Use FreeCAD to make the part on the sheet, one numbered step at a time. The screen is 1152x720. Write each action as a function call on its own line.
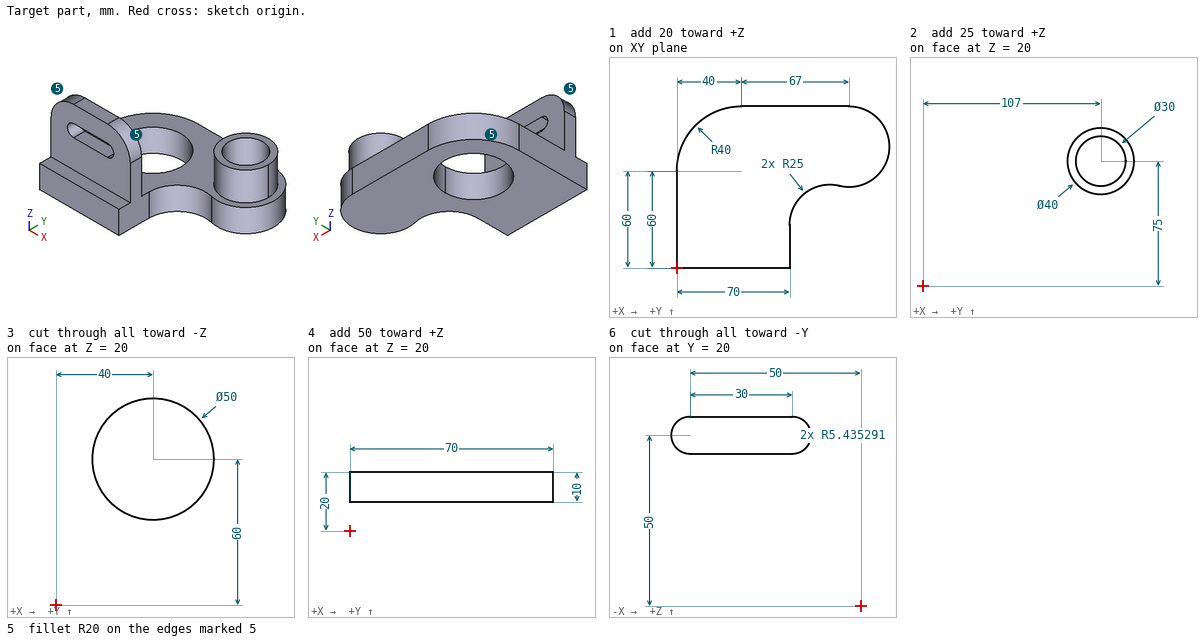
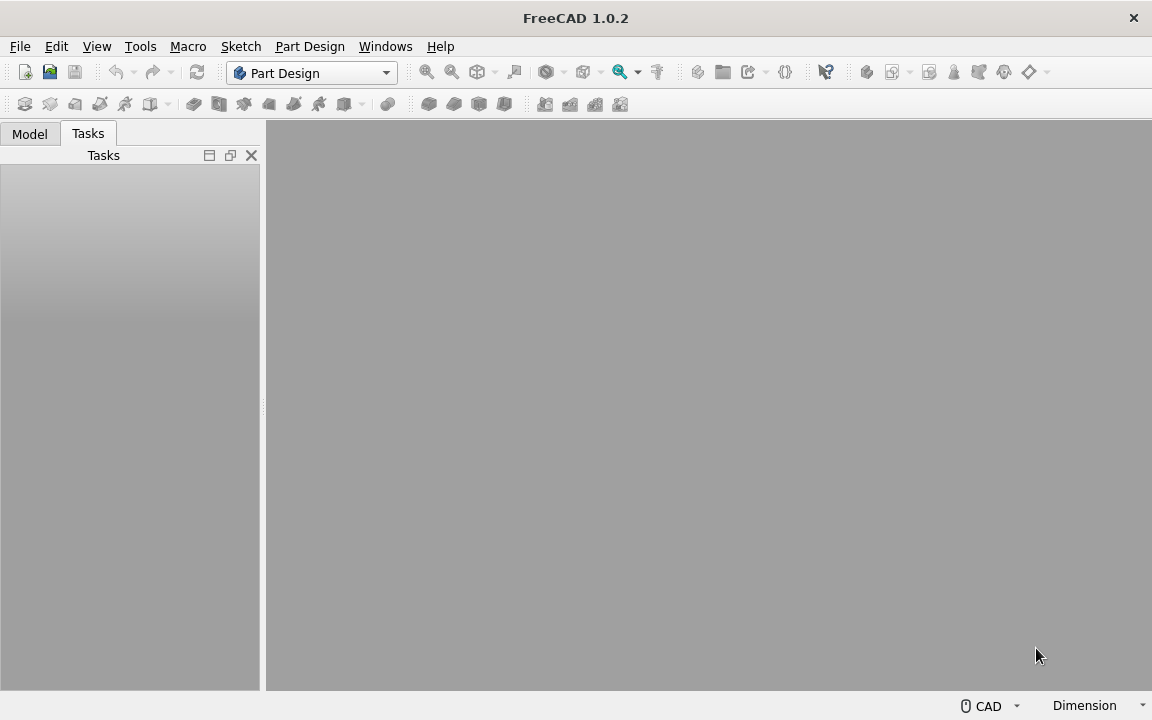
click(25, 72)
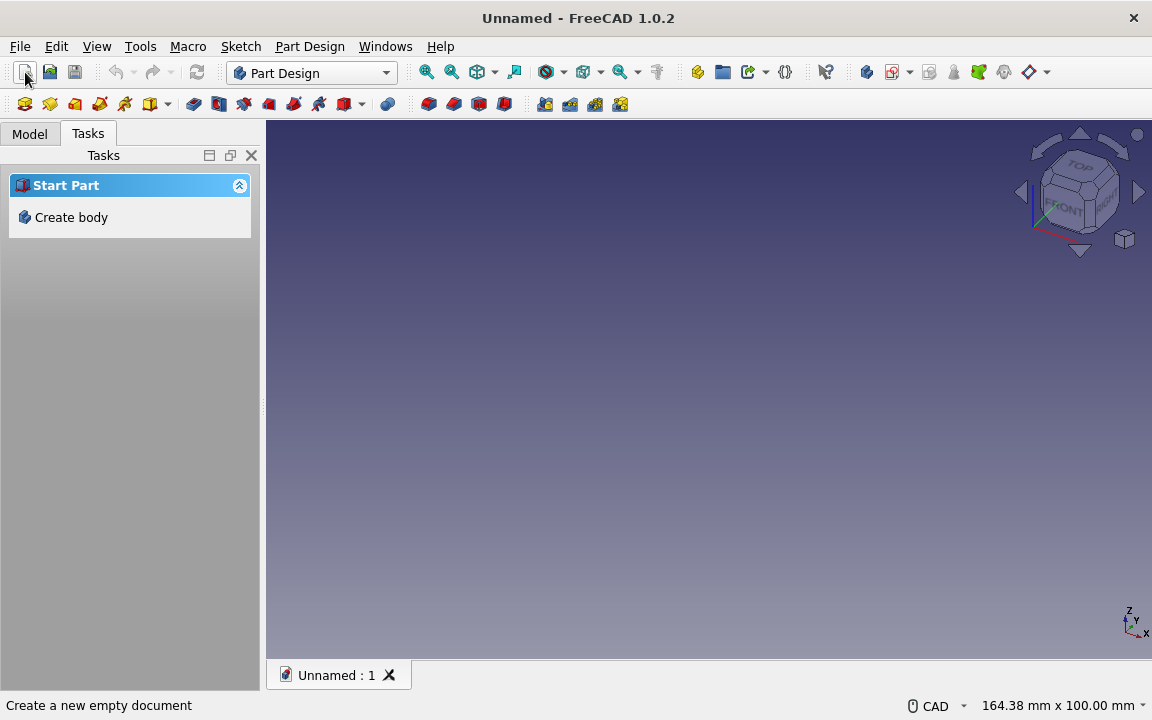
click(892, 72)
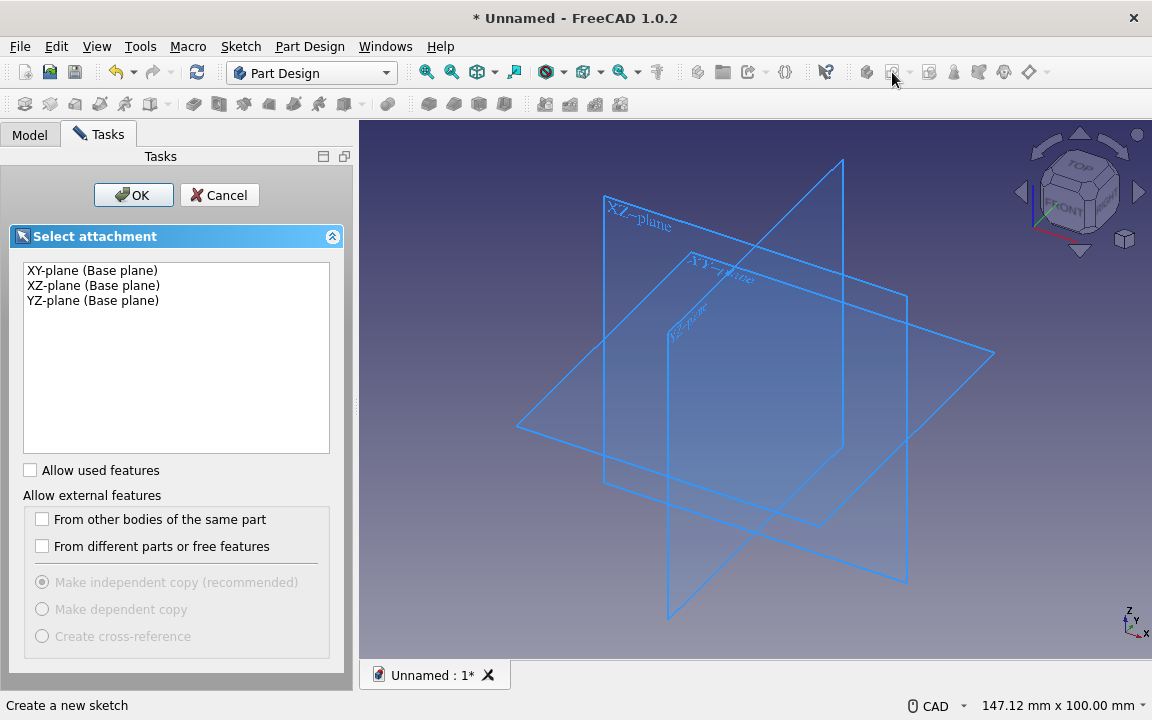
click(84, 270)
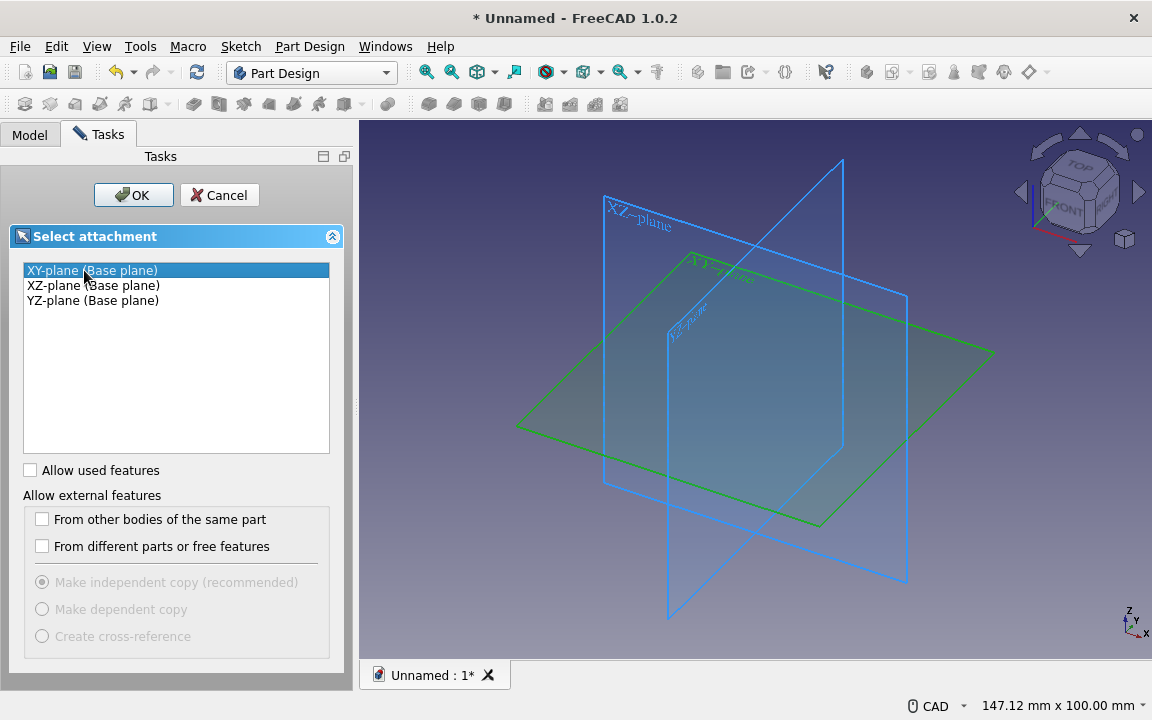
click(134, 195)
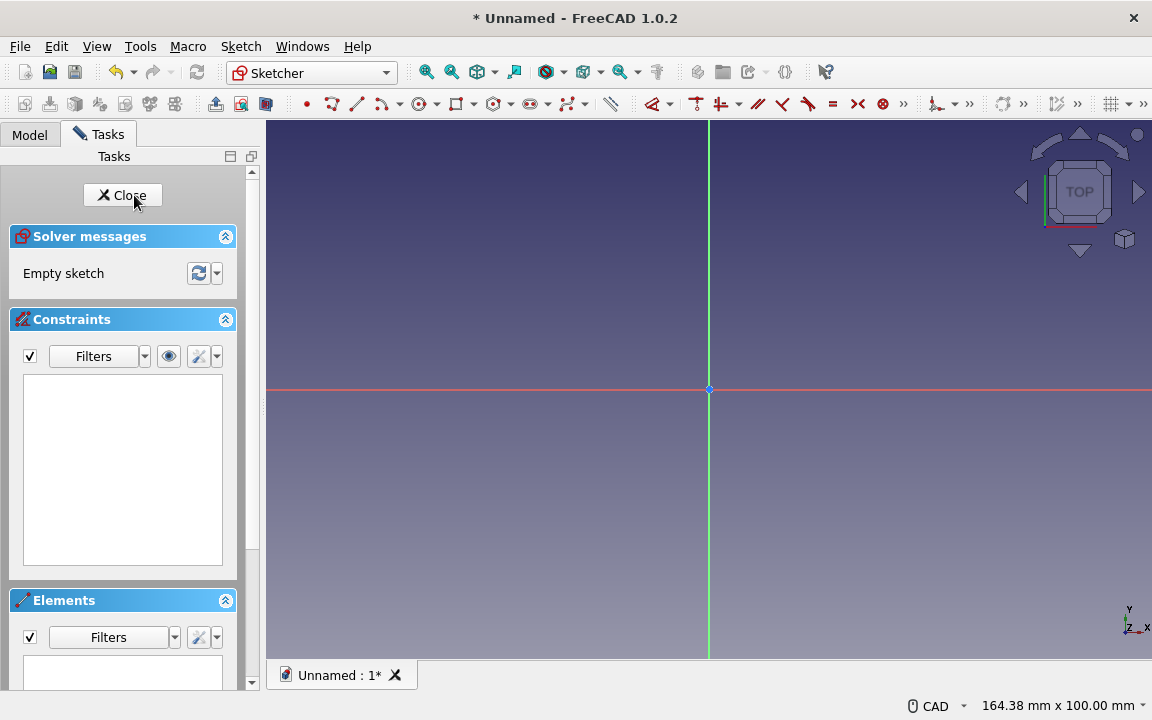
scroll(294, 631, down, 3)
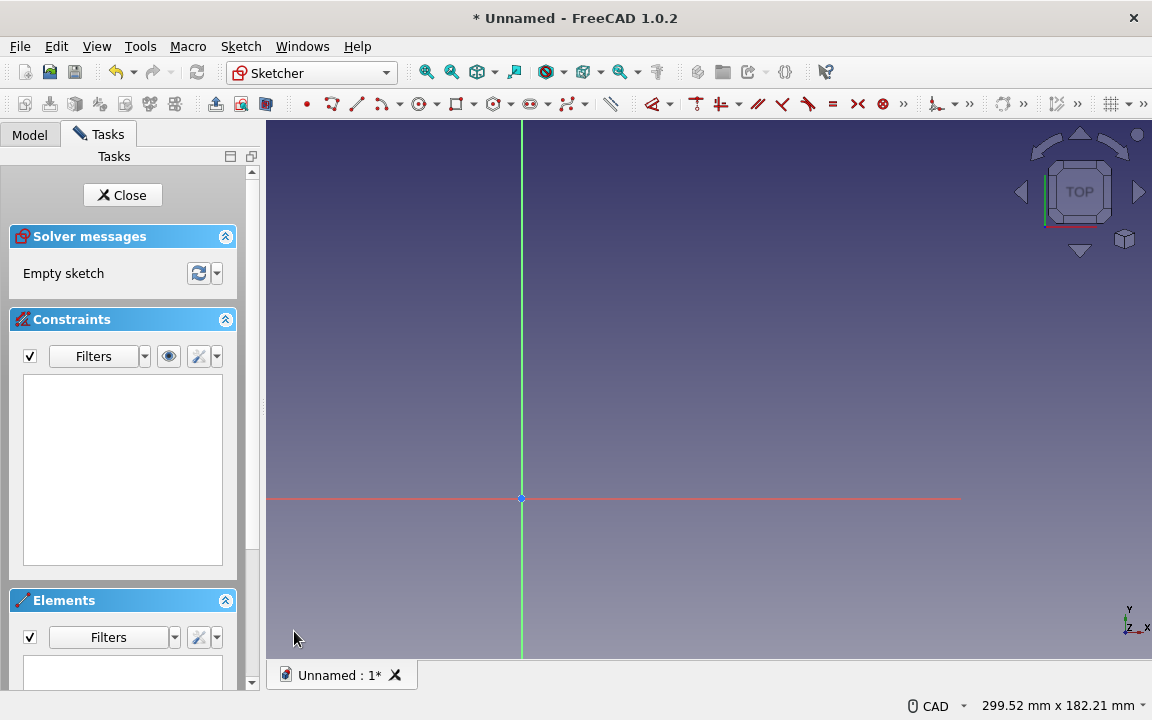
click(357, 104)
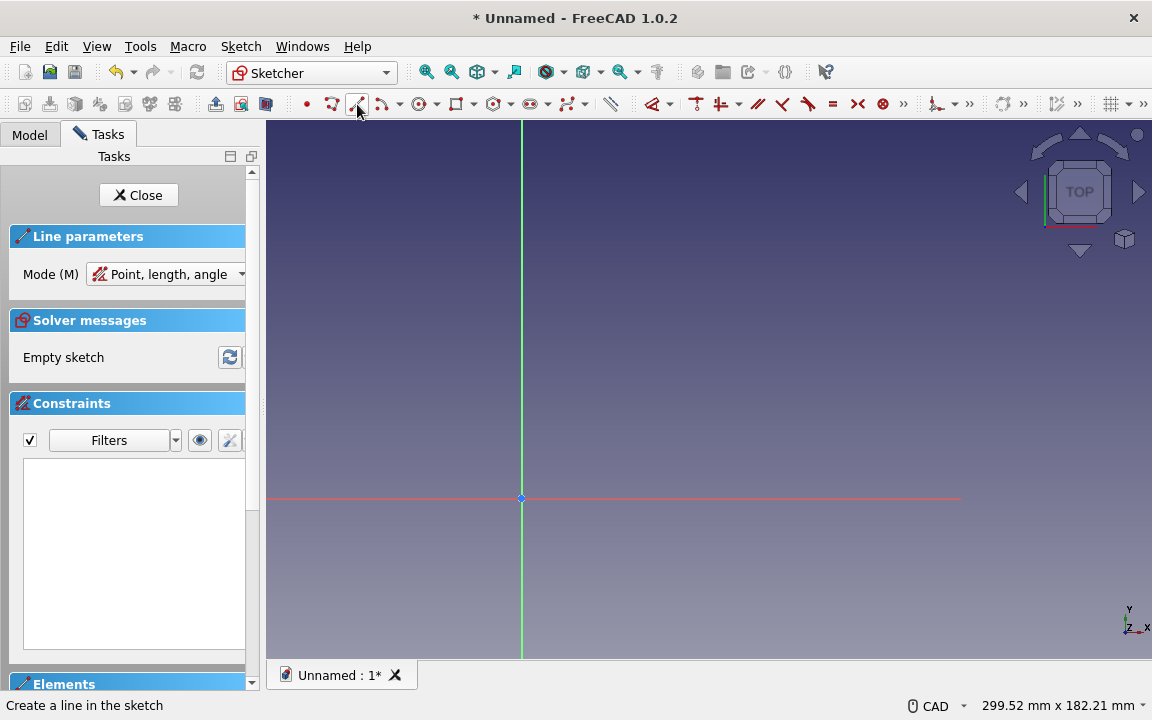
click(838, 203)
click(640, 203)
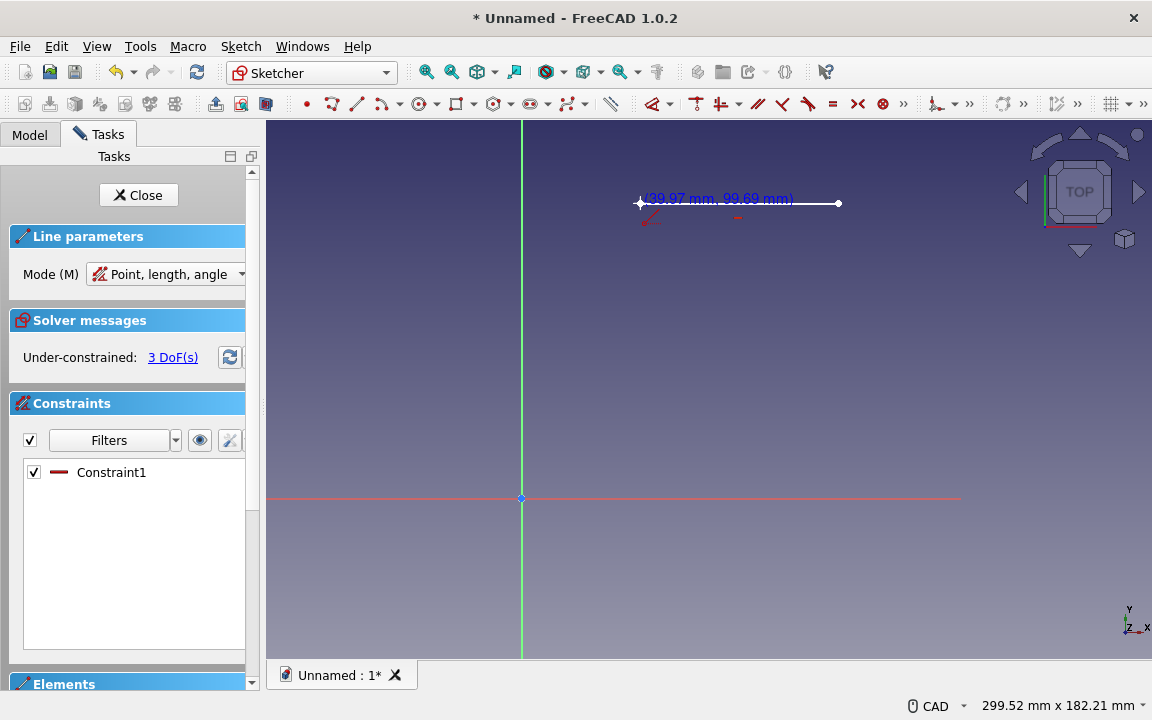
click(332, 104)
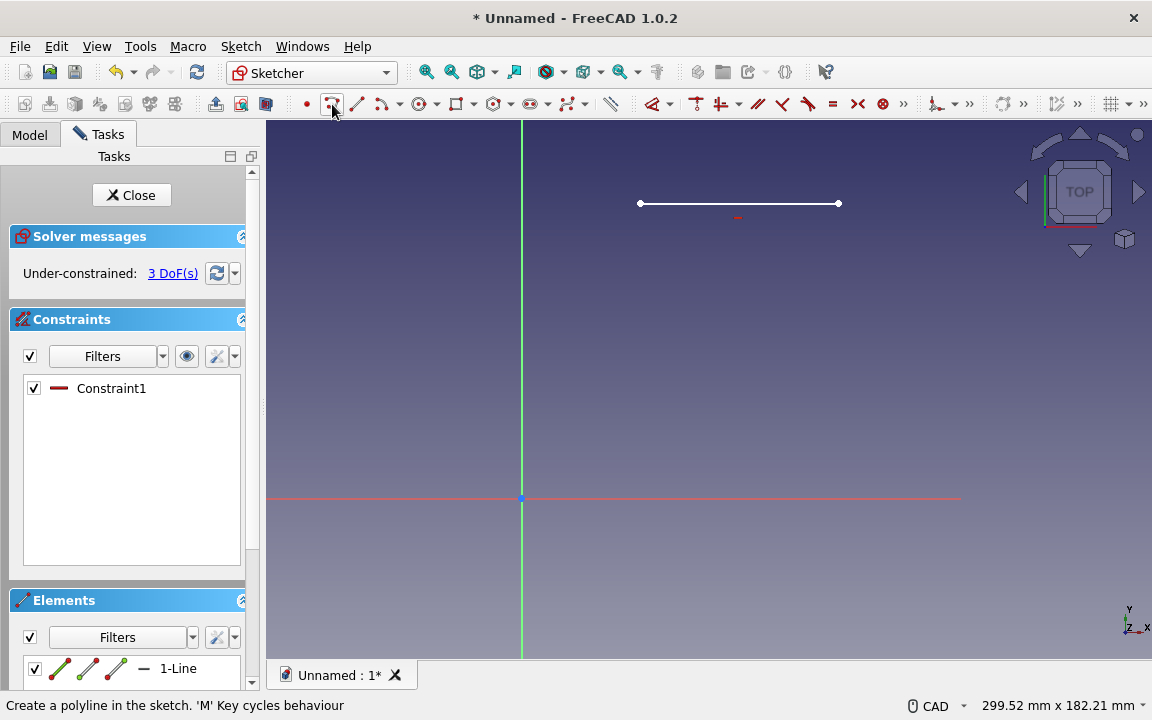
click(522, 321)
click(522, 499)
click(729, 490)
click(729, 421)
right_click(729, 421)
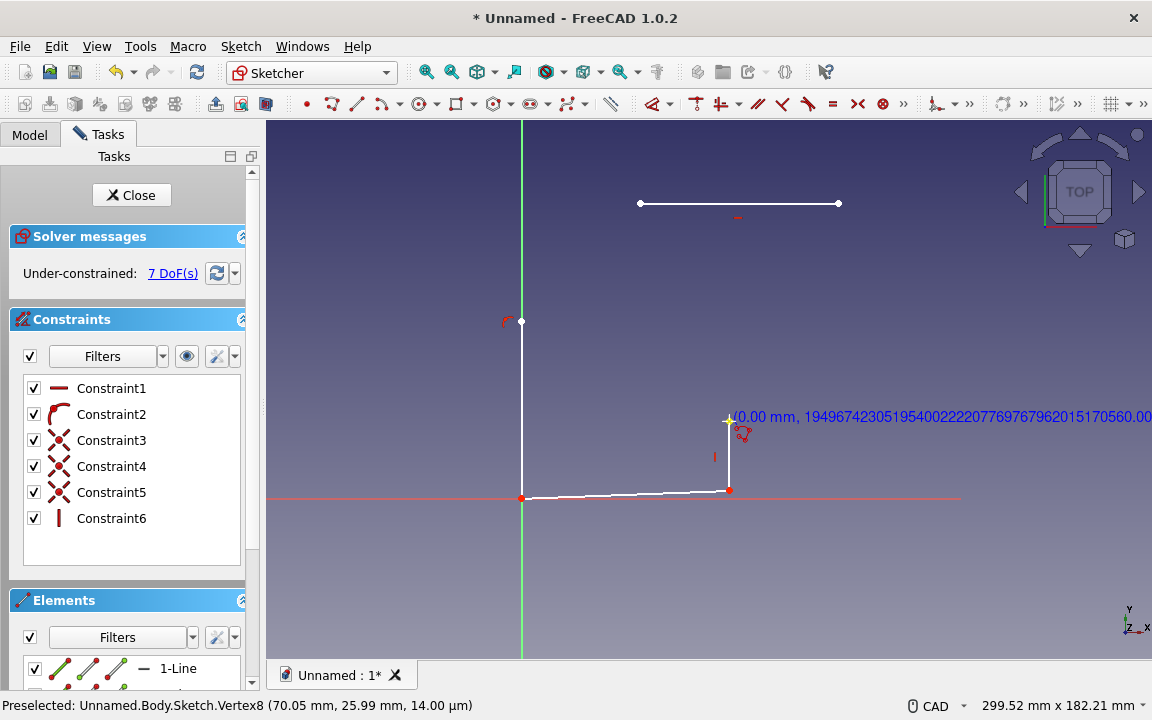
key(g)
key(3)
key(a)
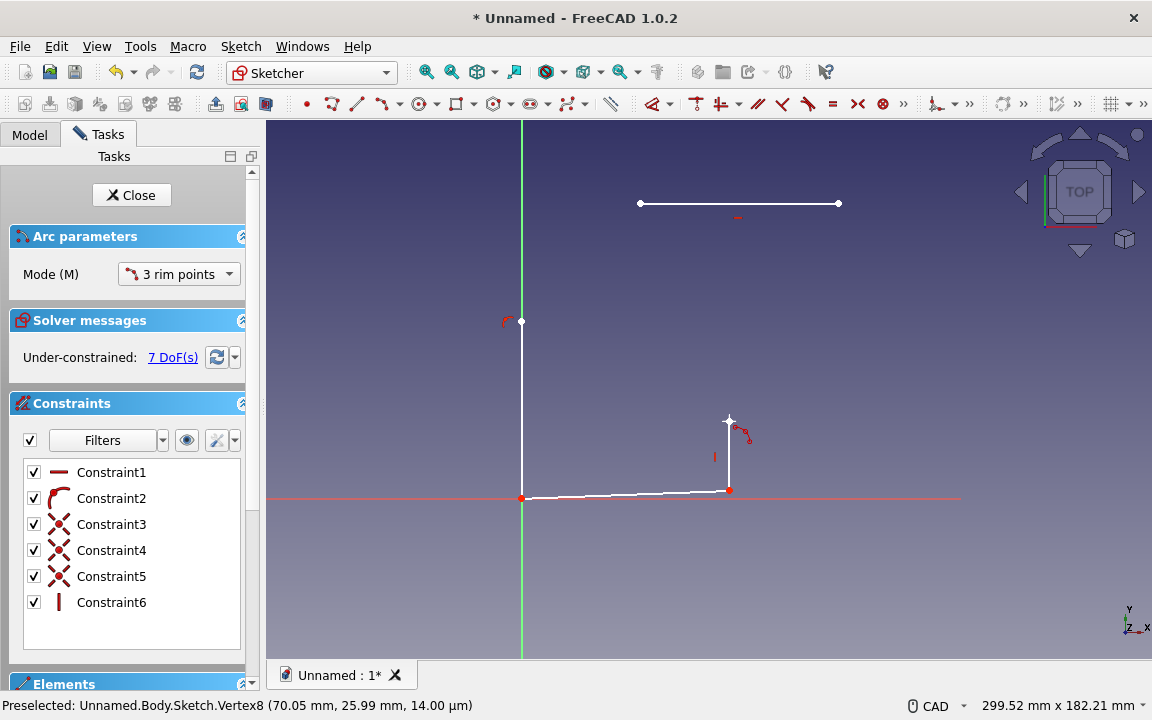
click(640, 204)
click(522, 322)
click(556, 238)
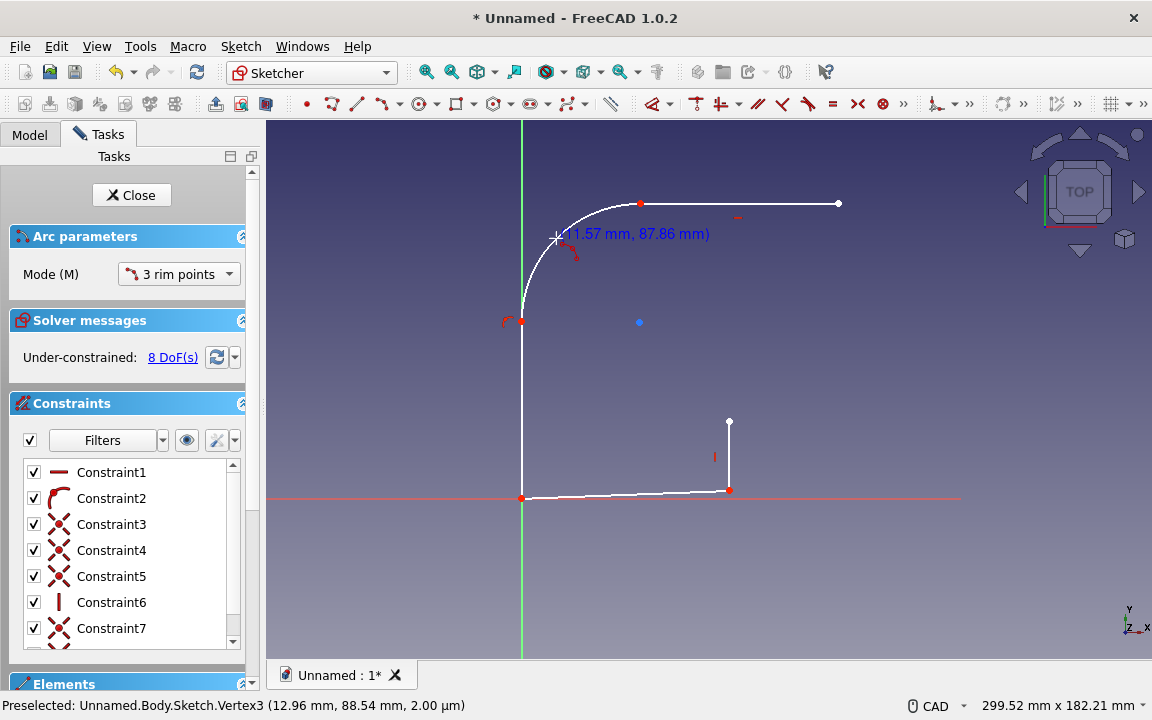
click(729, 422)
click(821, 349)
click(757, 362)